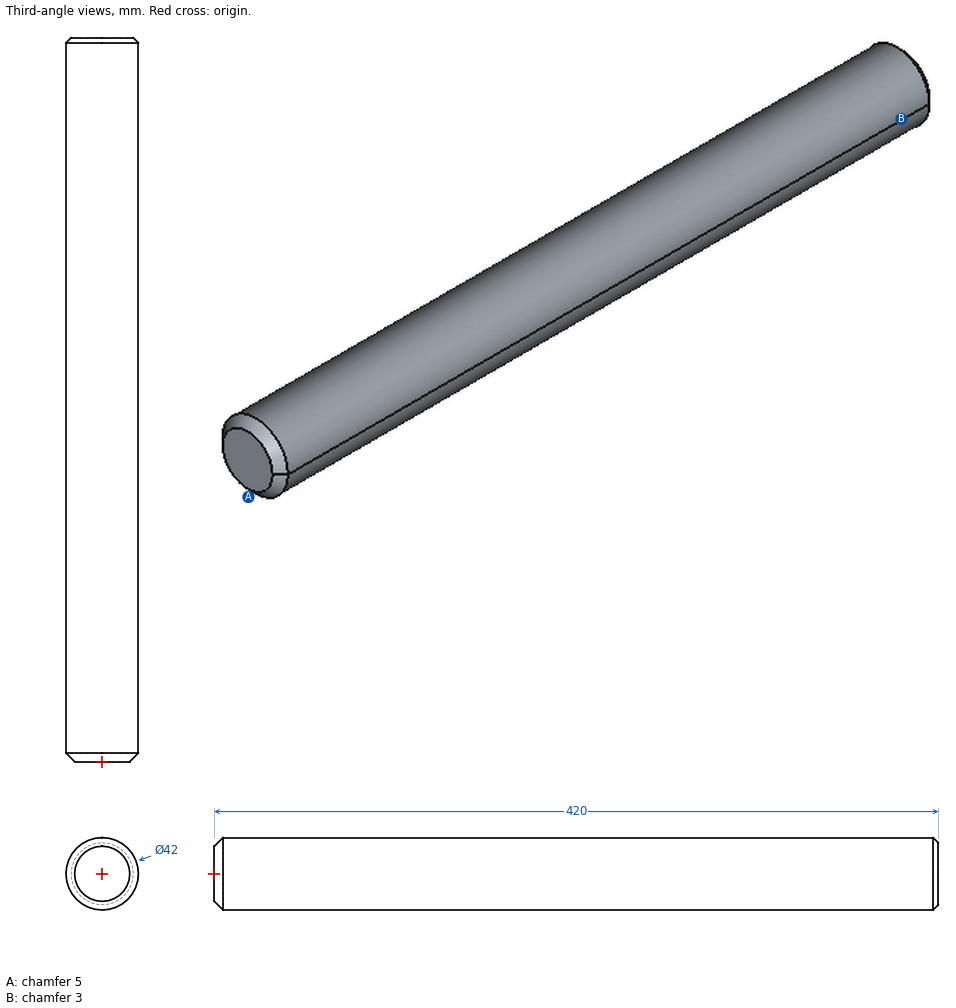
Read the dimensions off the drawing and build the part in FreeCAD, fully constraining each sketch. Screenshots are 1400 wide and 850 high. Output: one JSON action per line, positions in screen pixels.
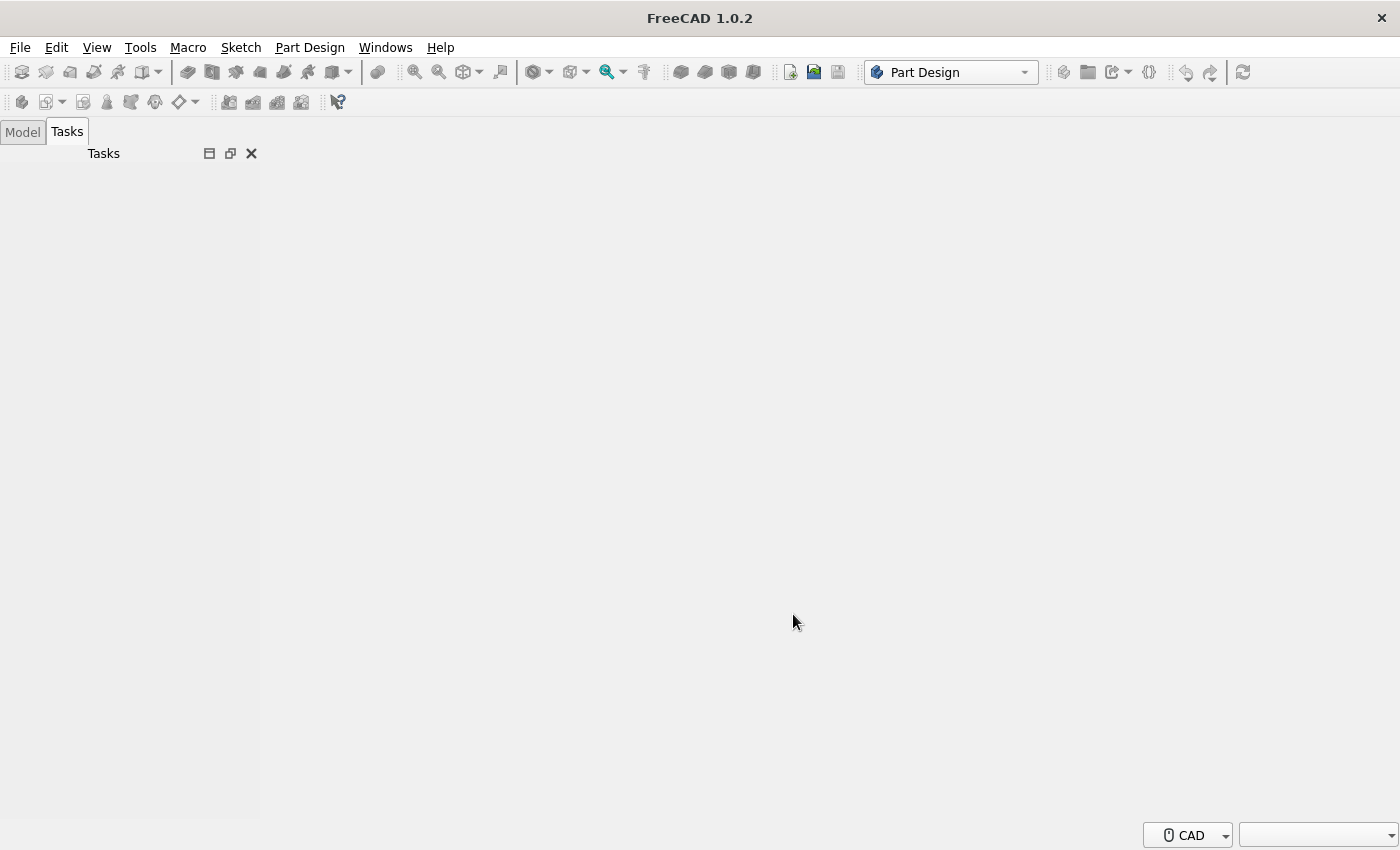
{"action": "left_click", "coordinate": [790, 72]}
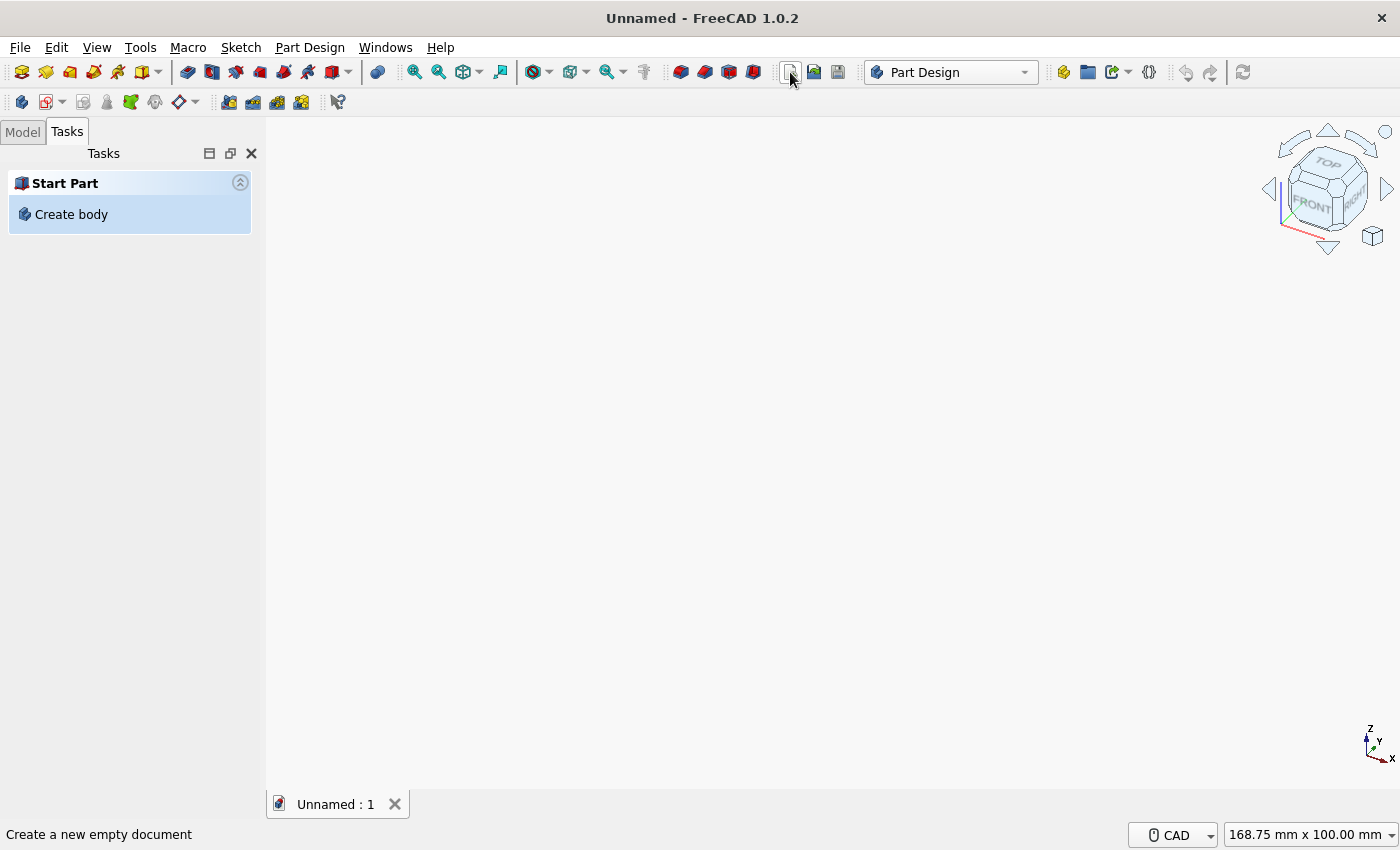
{"action": "left_click", "coordinate": [46, 102]}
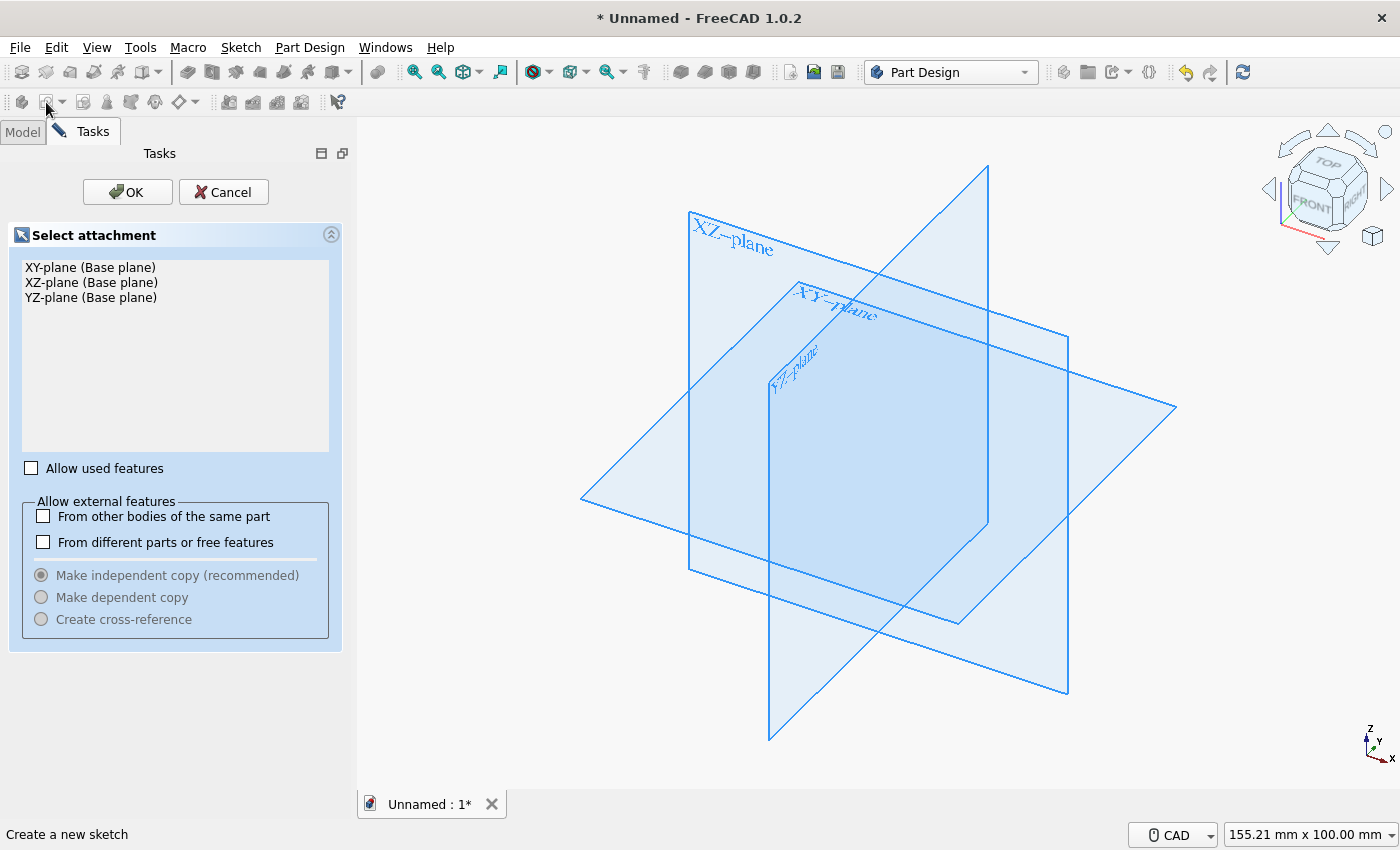
{"action": "left_click", "coordinate": [82, 282]}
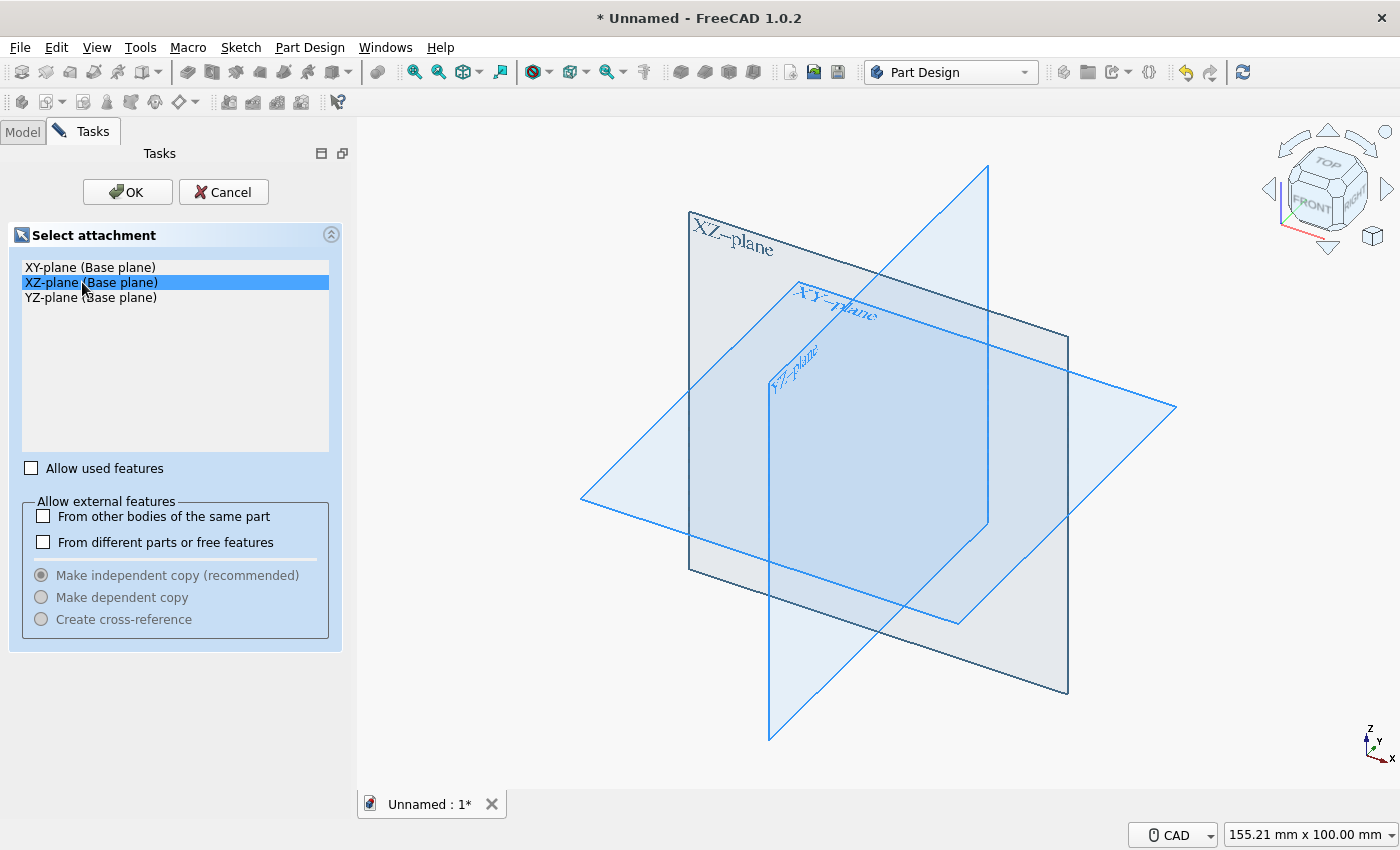
{"action": "left_click", "coordinate": [128, 192]}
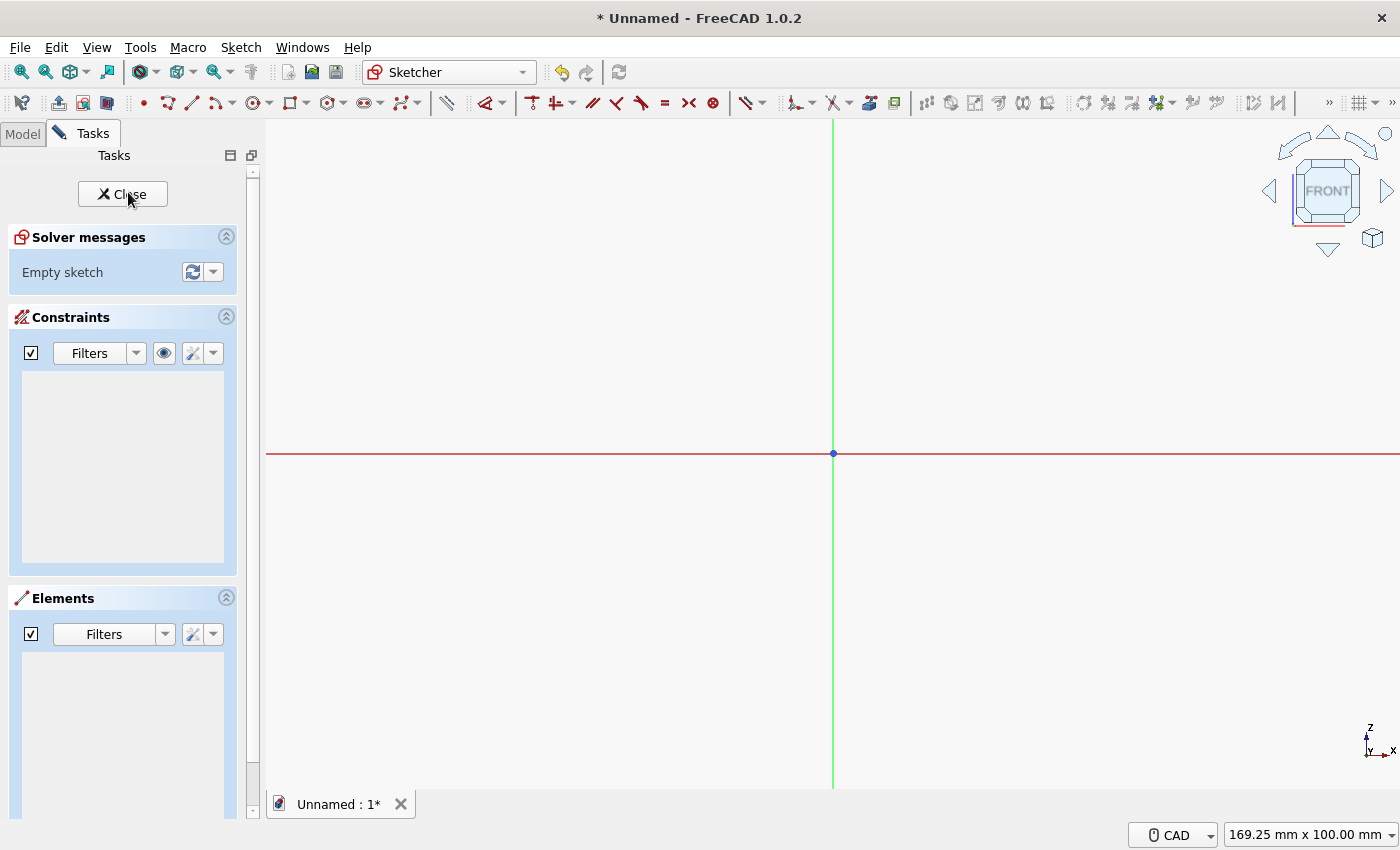
{"action": "scroll", "coordinate": [972, 454], "scroll_direction": "up", "scroll_amount": 2}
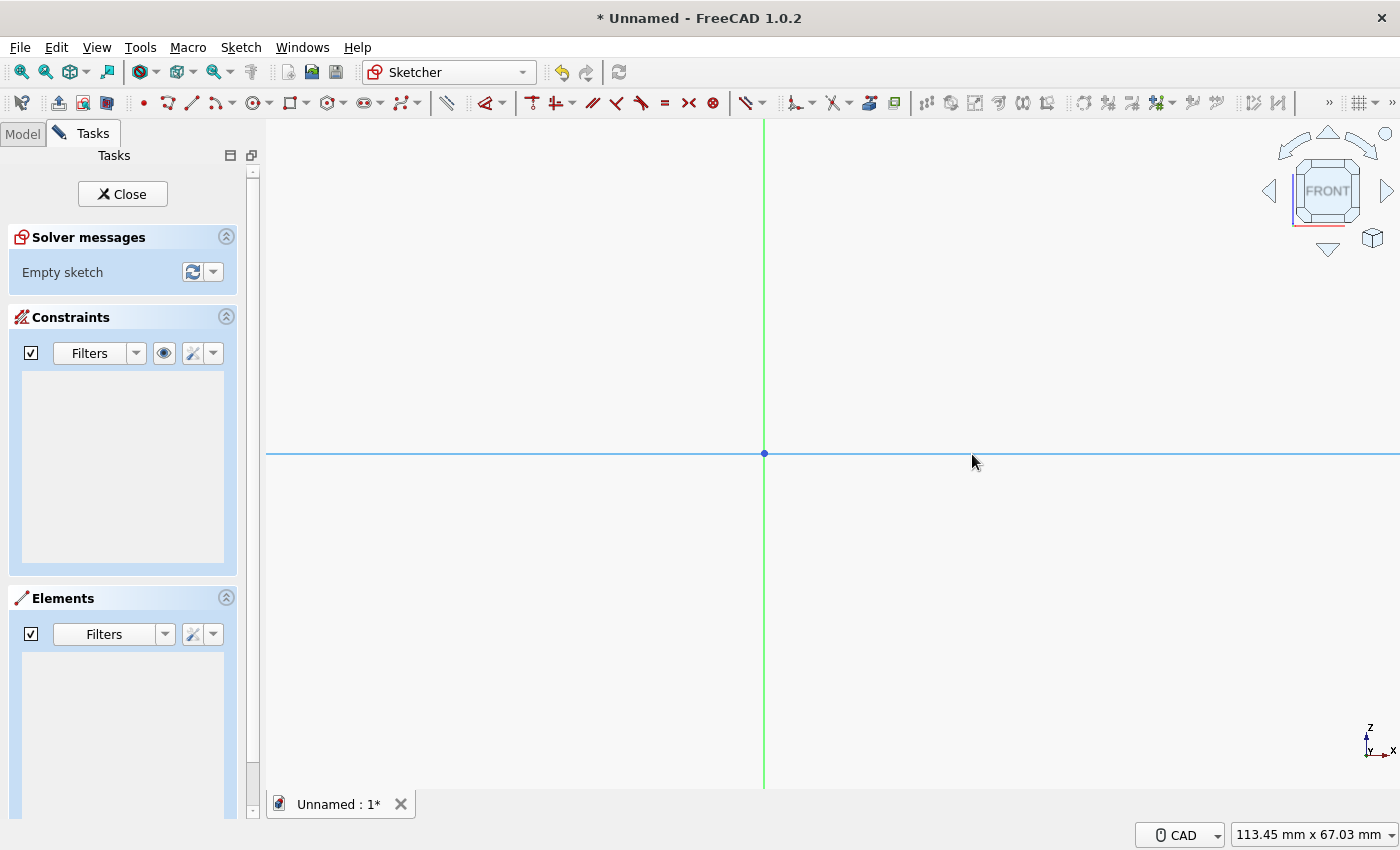
{"action": "left_click", "coordinate": [254, 104]}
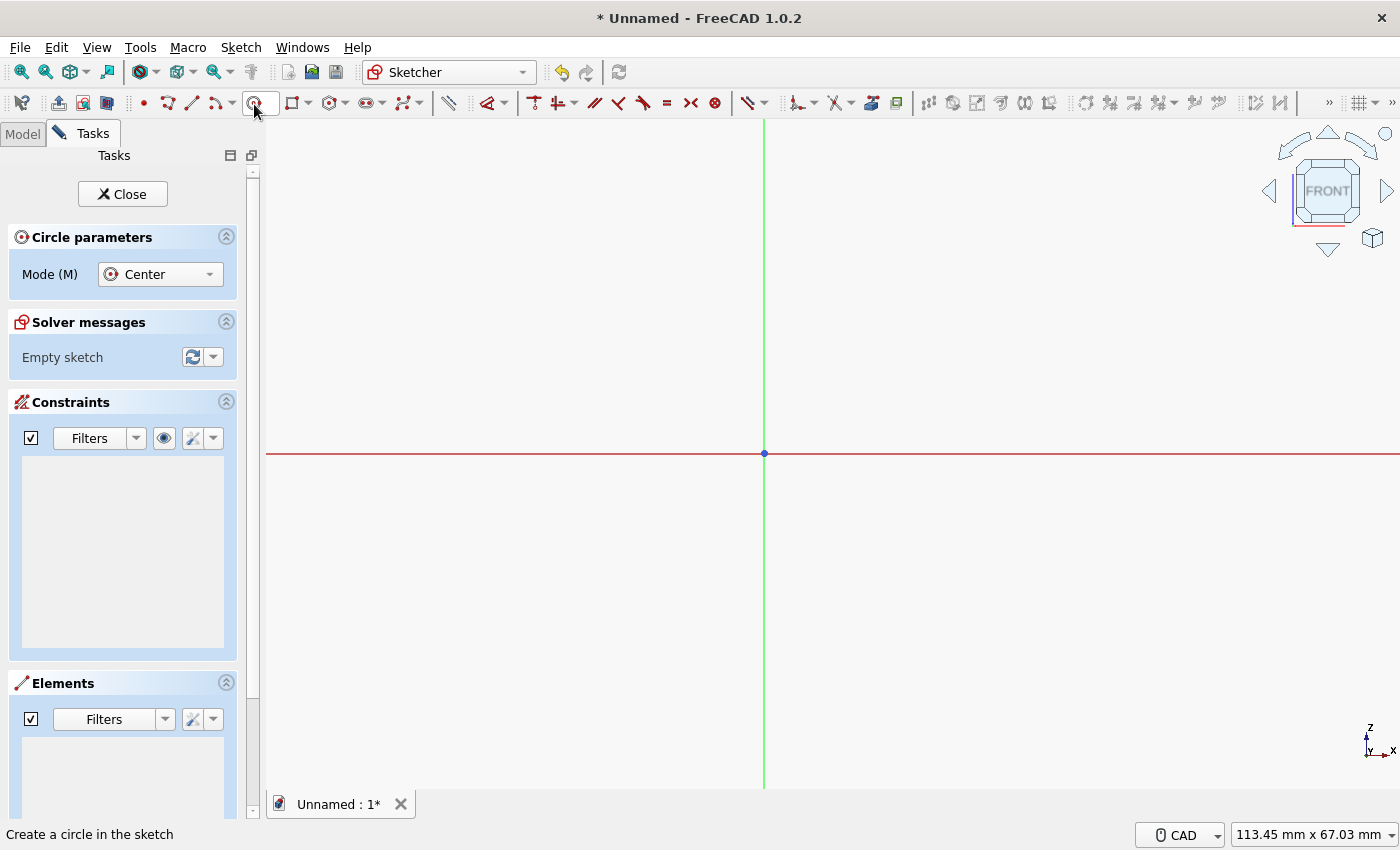
{"action": "left_click", "coordinate": [764, 454]}
{"action": "mouse_move", "coordinate": [913, 305]}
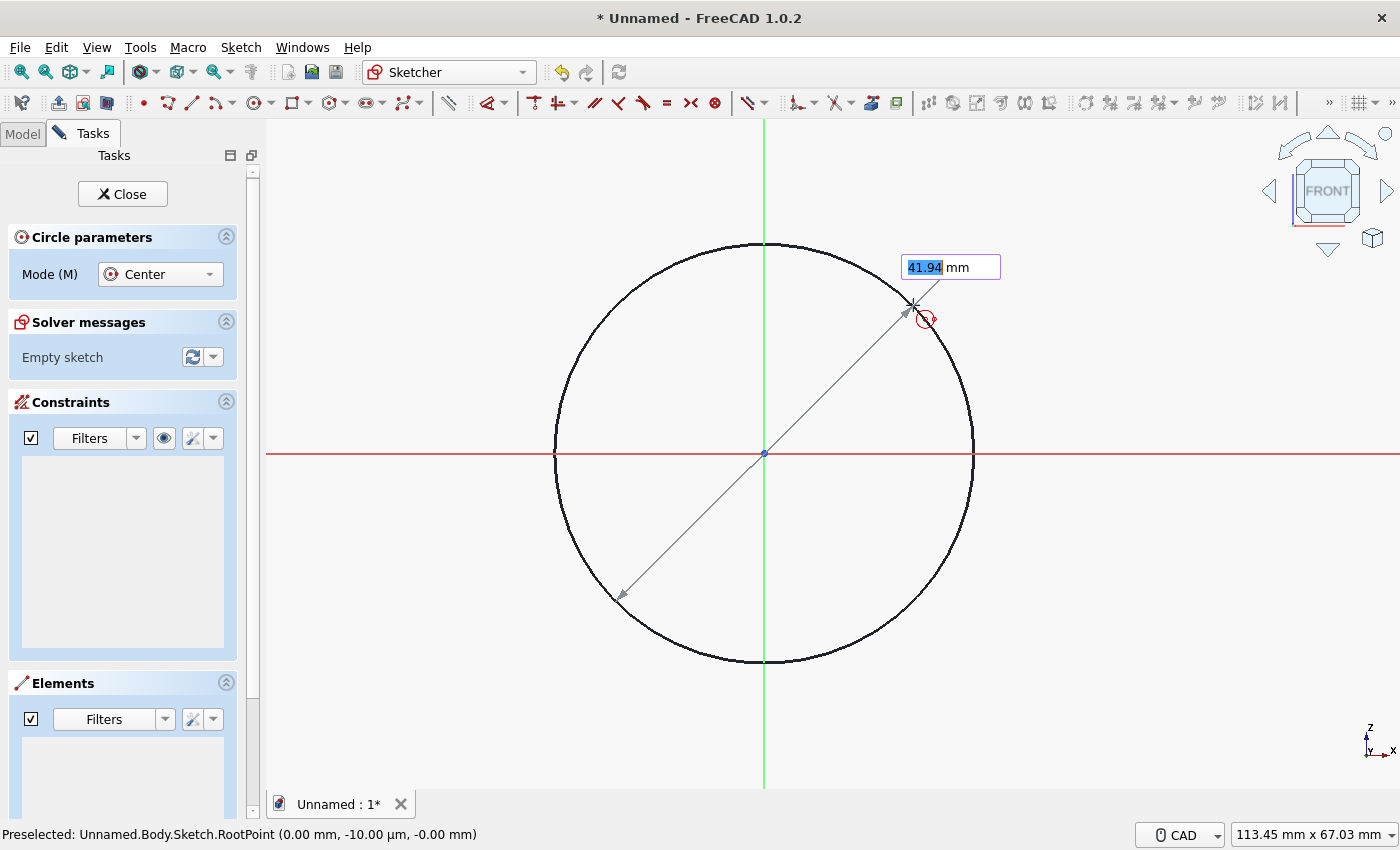
{"action": "type", "text": "42"}
{"action": "key", "text": "Return"}
{"action": "key", "text": "Escape"}